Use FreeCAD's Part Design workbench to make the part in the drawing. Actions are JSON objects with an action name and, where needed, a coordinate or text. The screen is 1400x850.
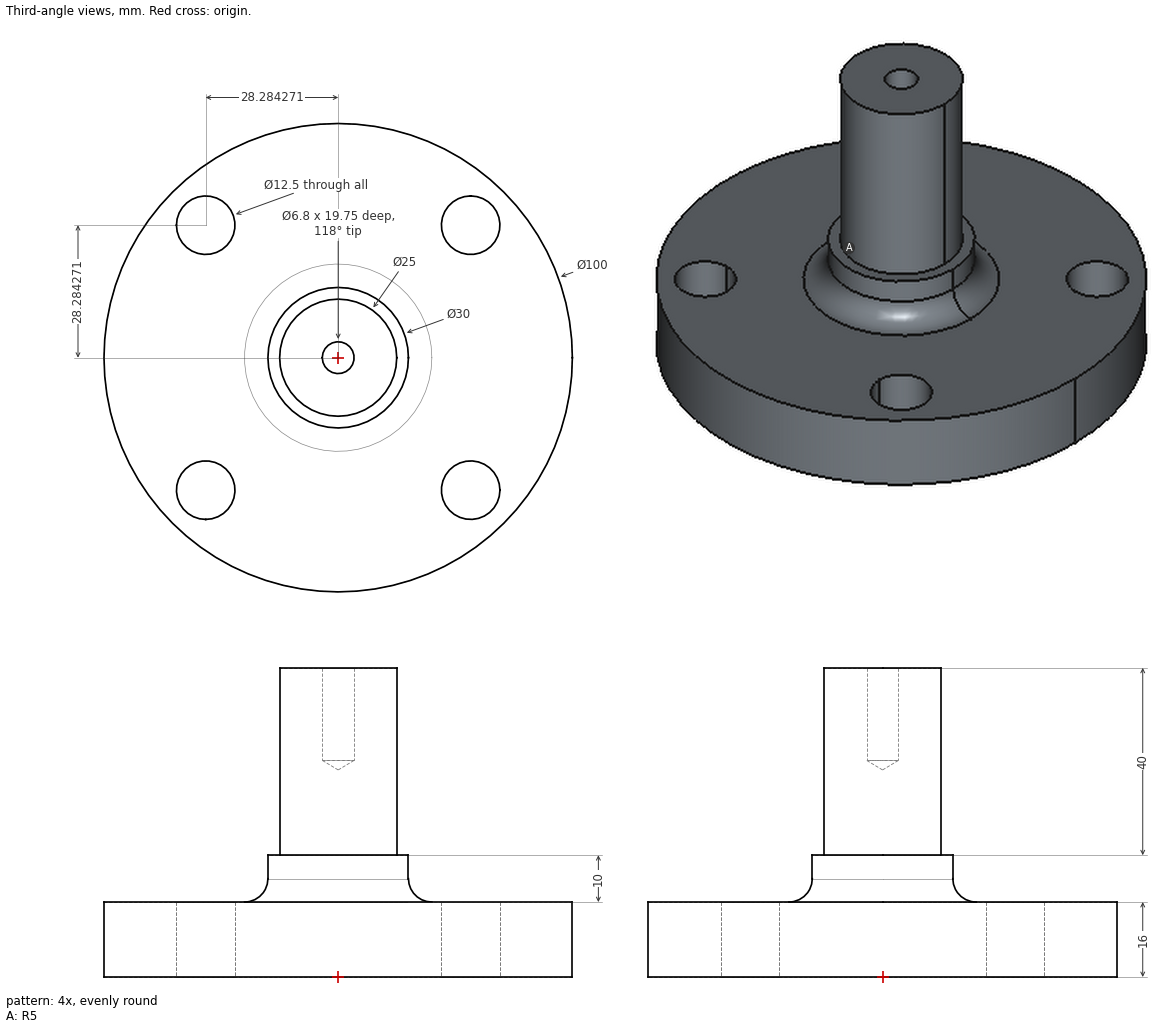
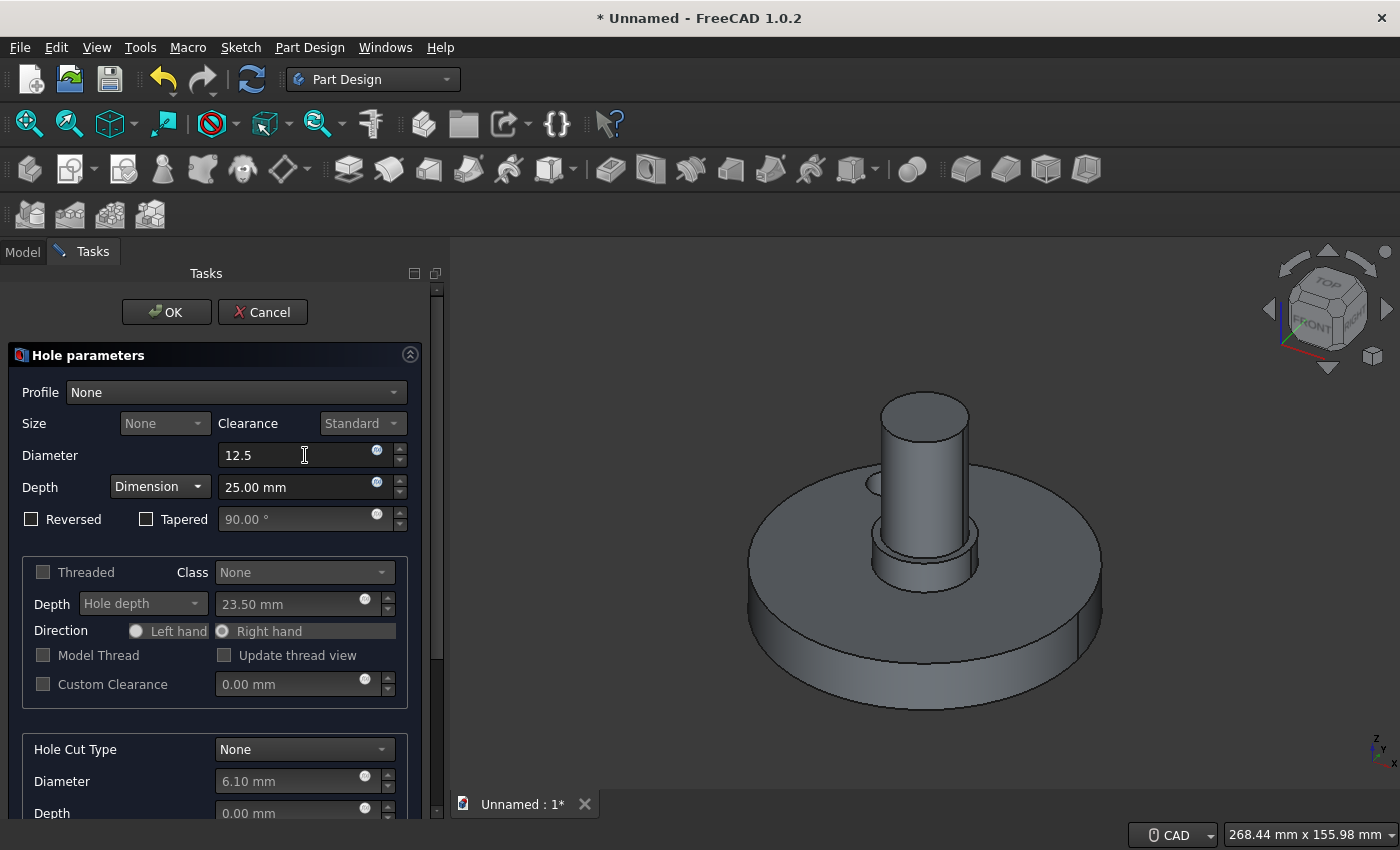
{"action": "left_click", "coordinate": [161, 486]}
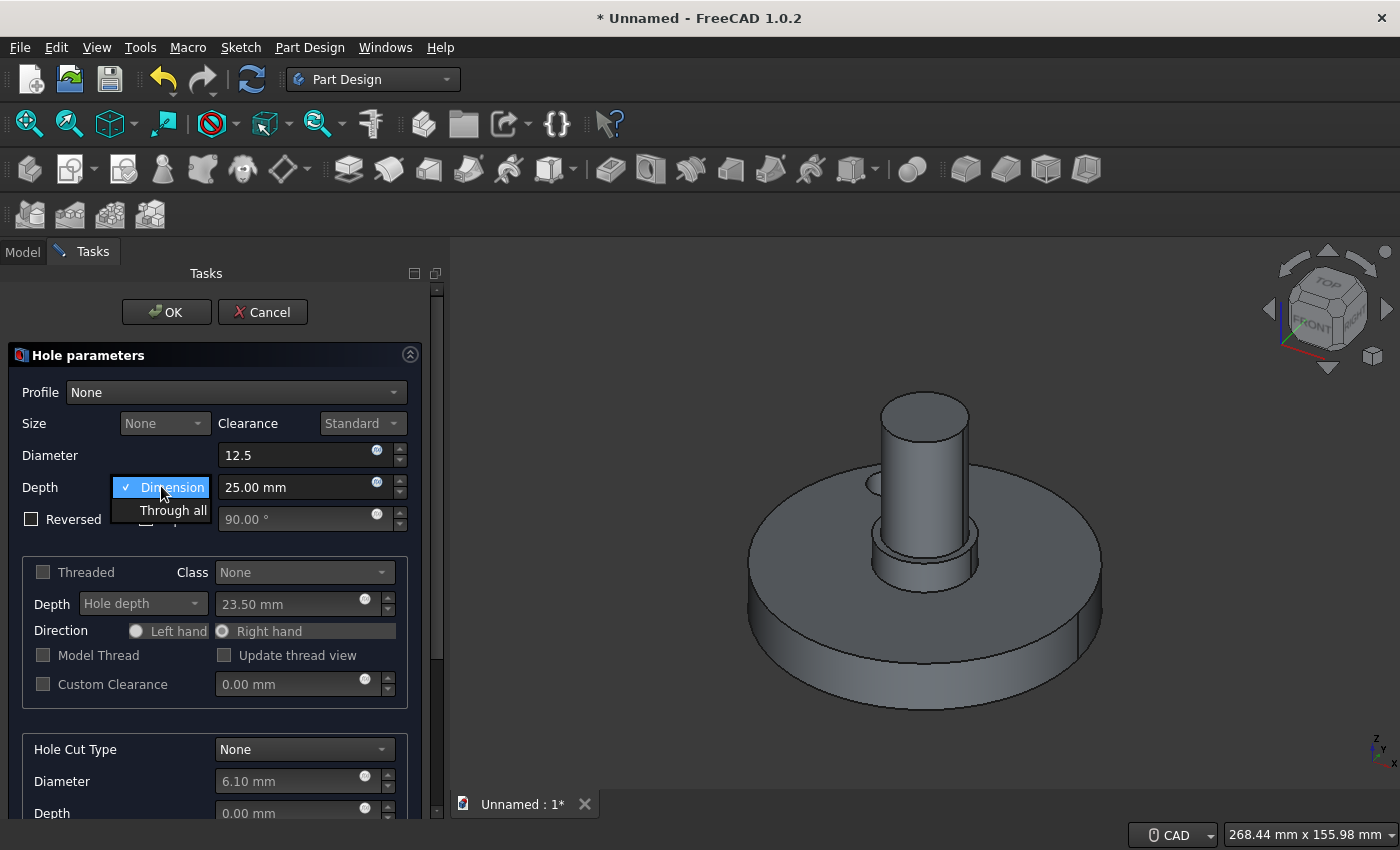
{"action": "left_click", "coordinate": [160, 510]}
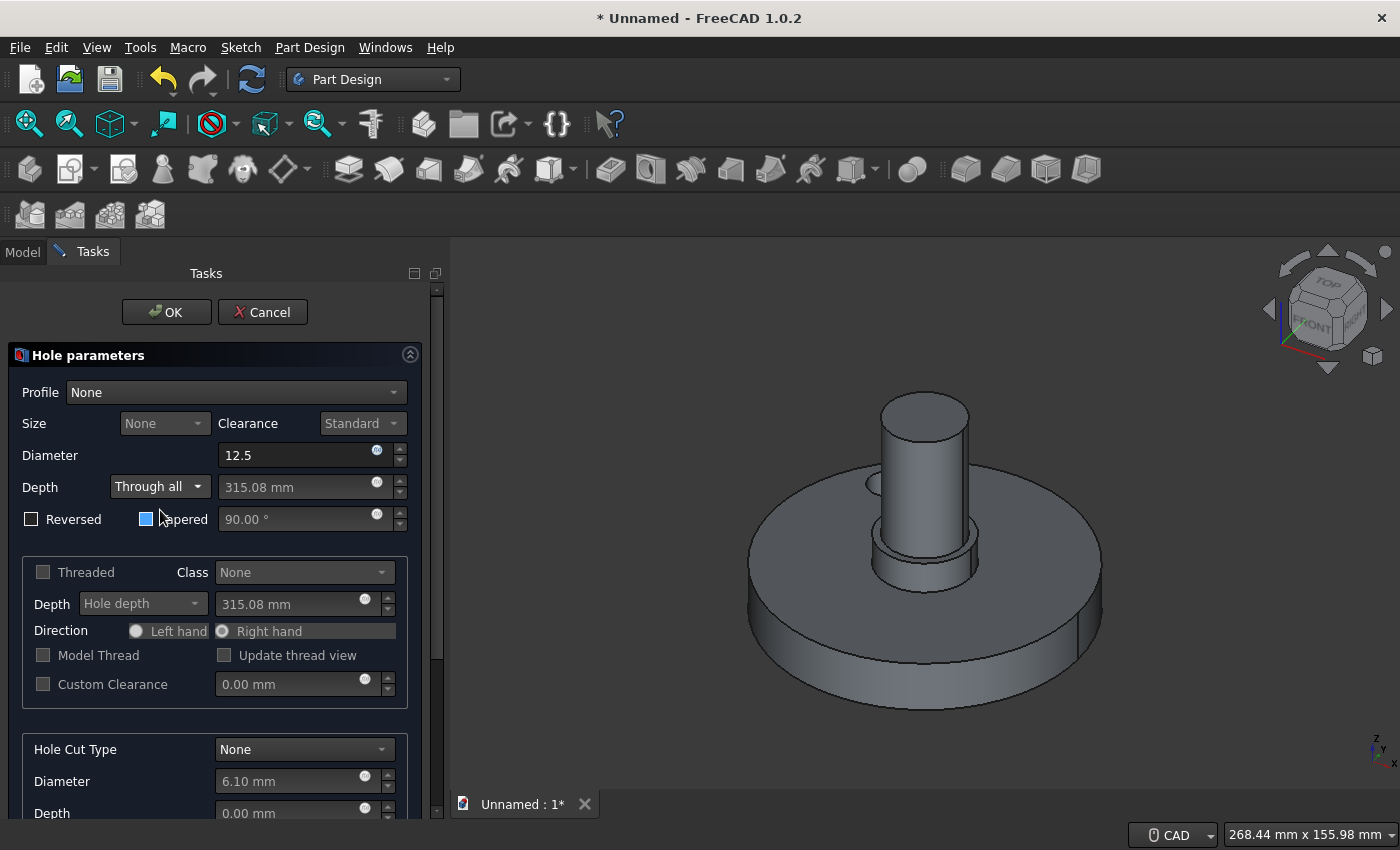
{"action": "left_click", "coordinate": [167, 312]}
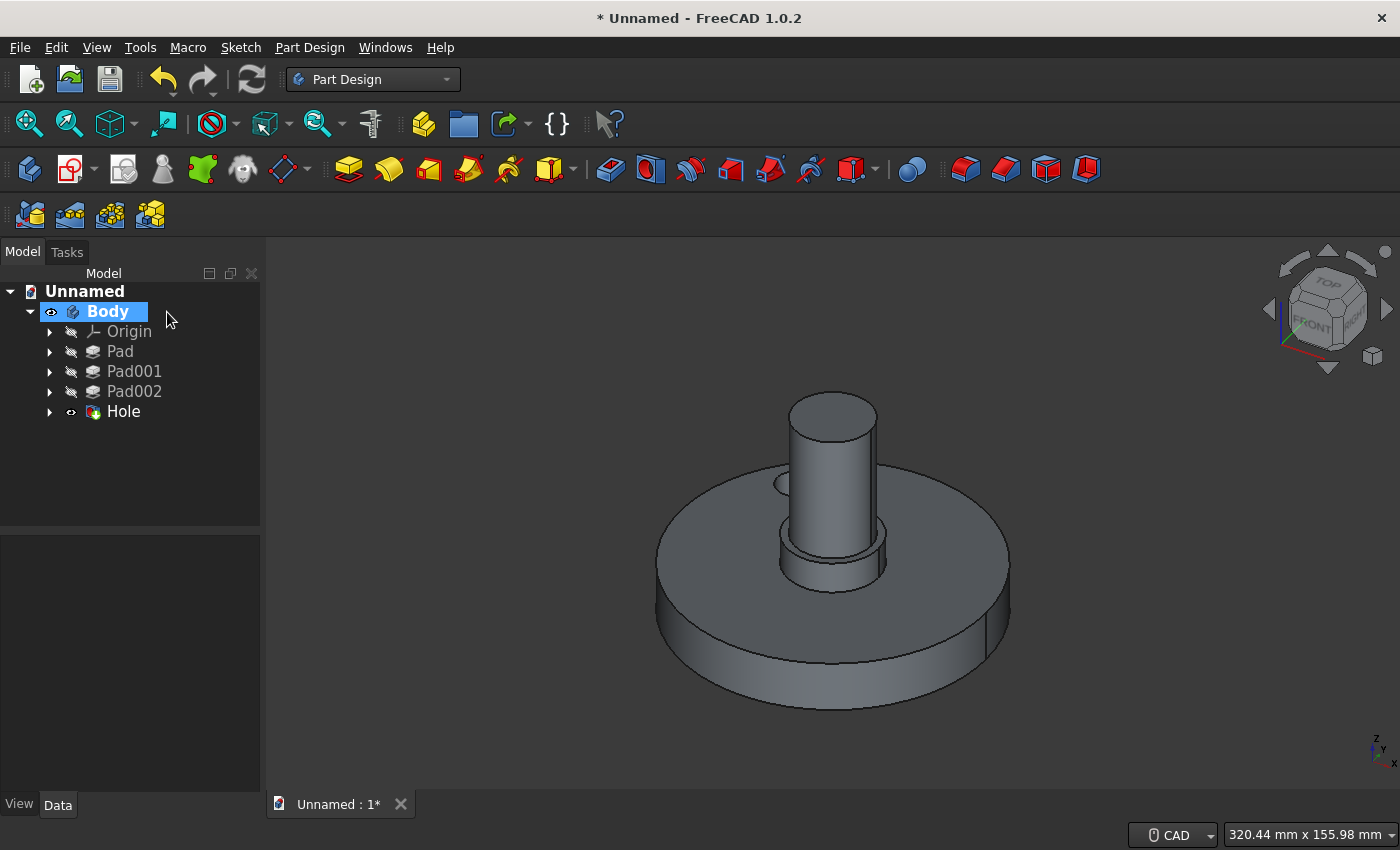
{"action": "left_click", "coordinate": [116, 412]}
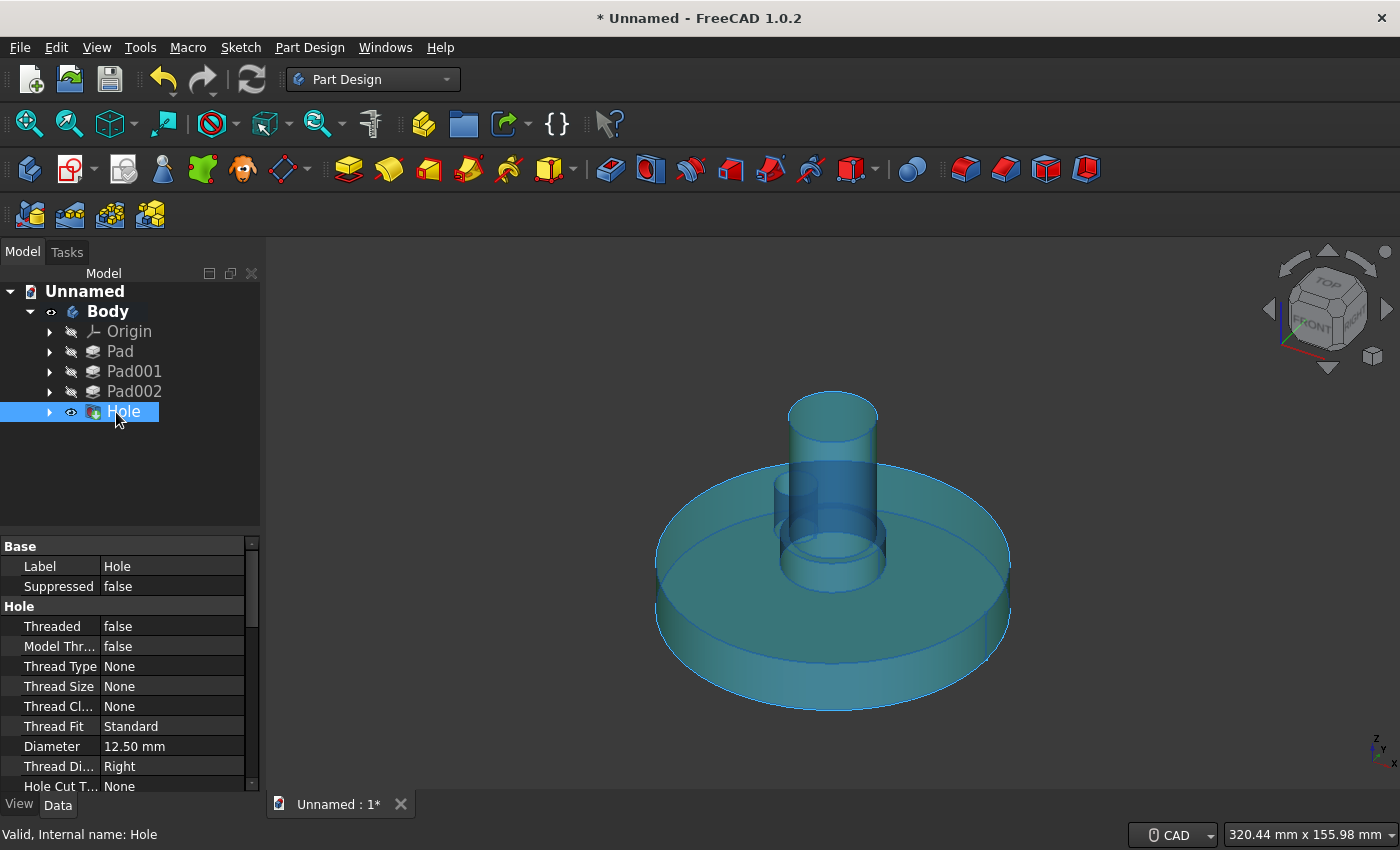
{"action": "left_click", "coordinate": [110, 214]}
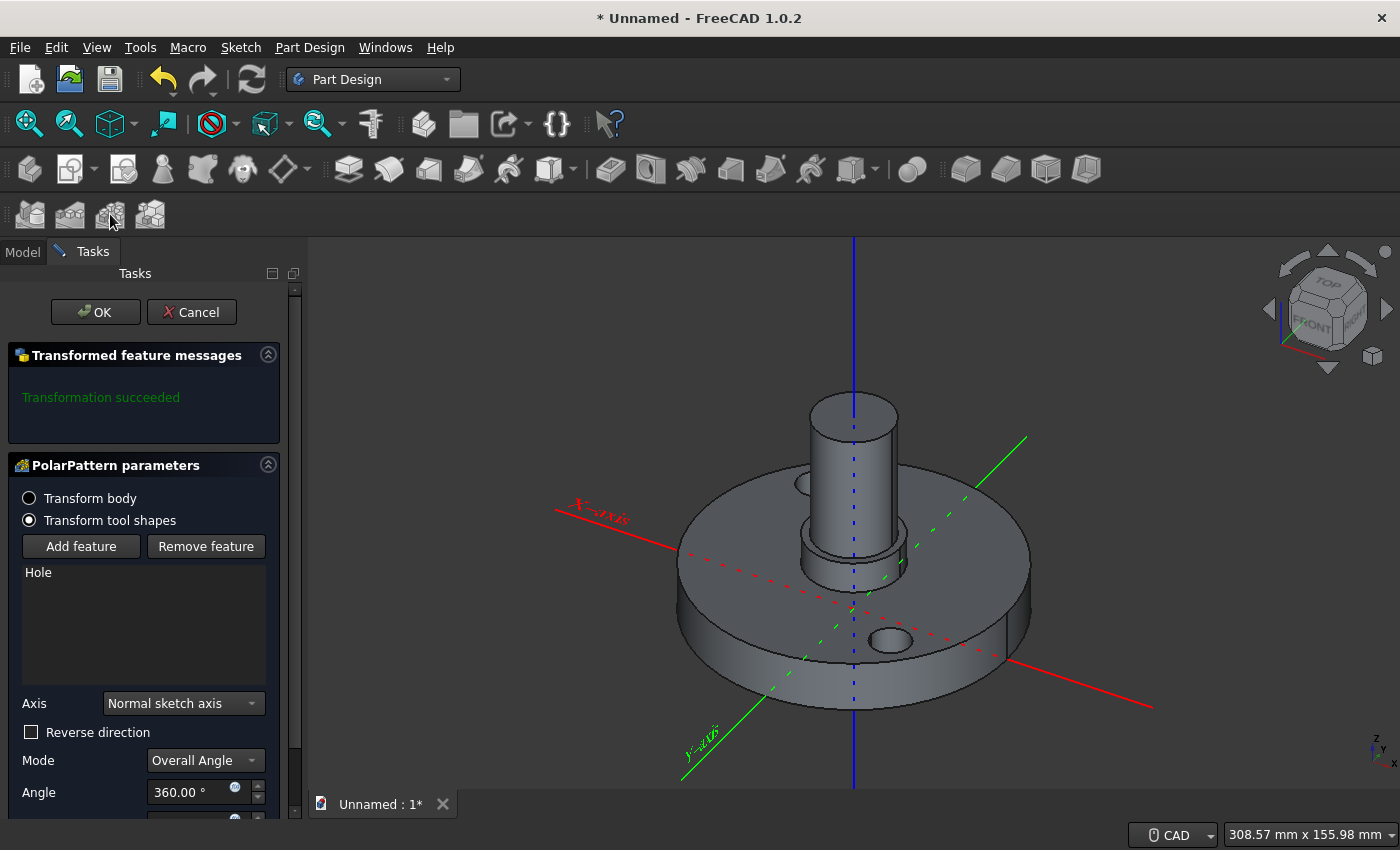
{"action": "left_click", "coordinate": [184, 704]}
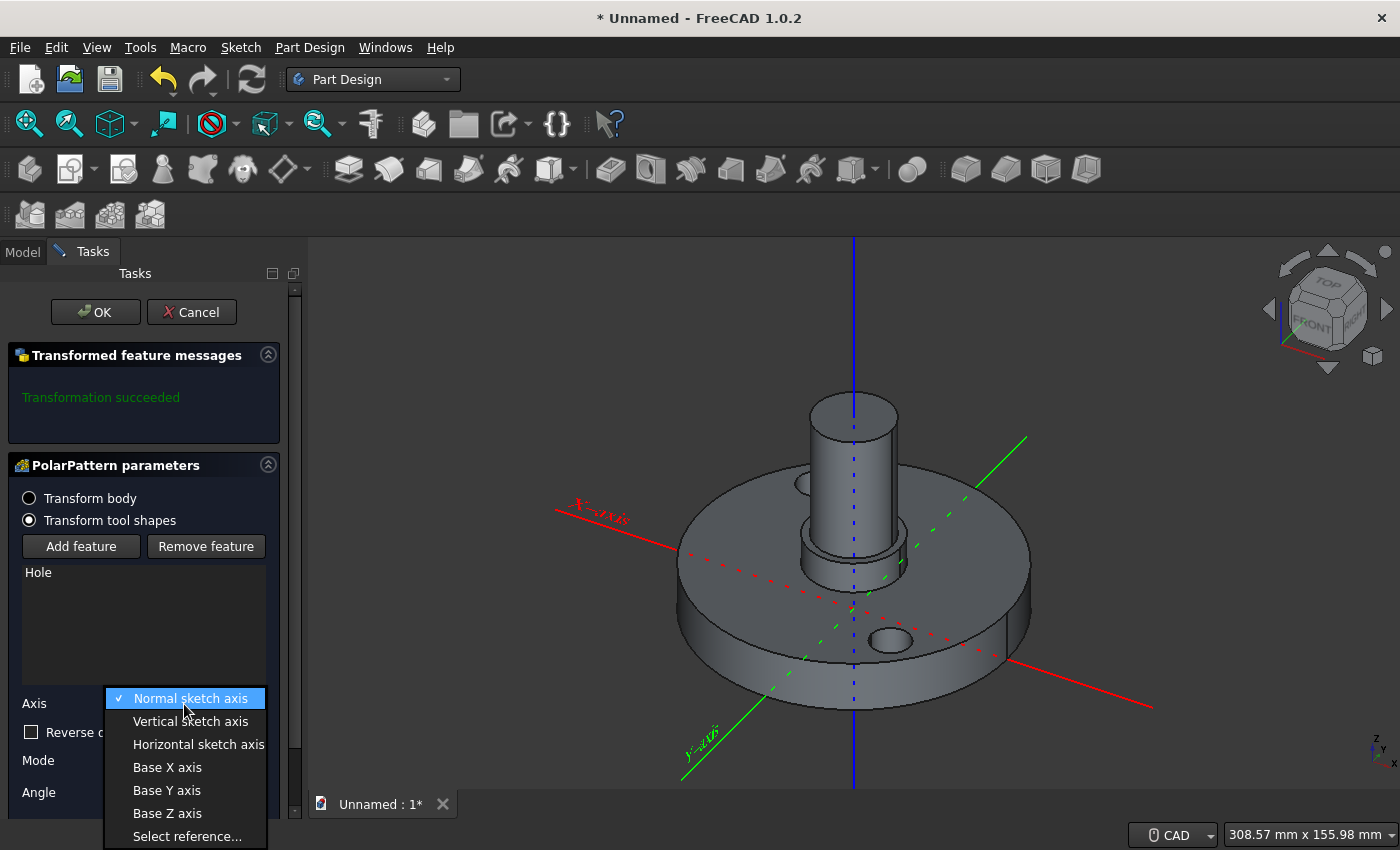
{"action": "left_click", "coordinate": [184, 814]}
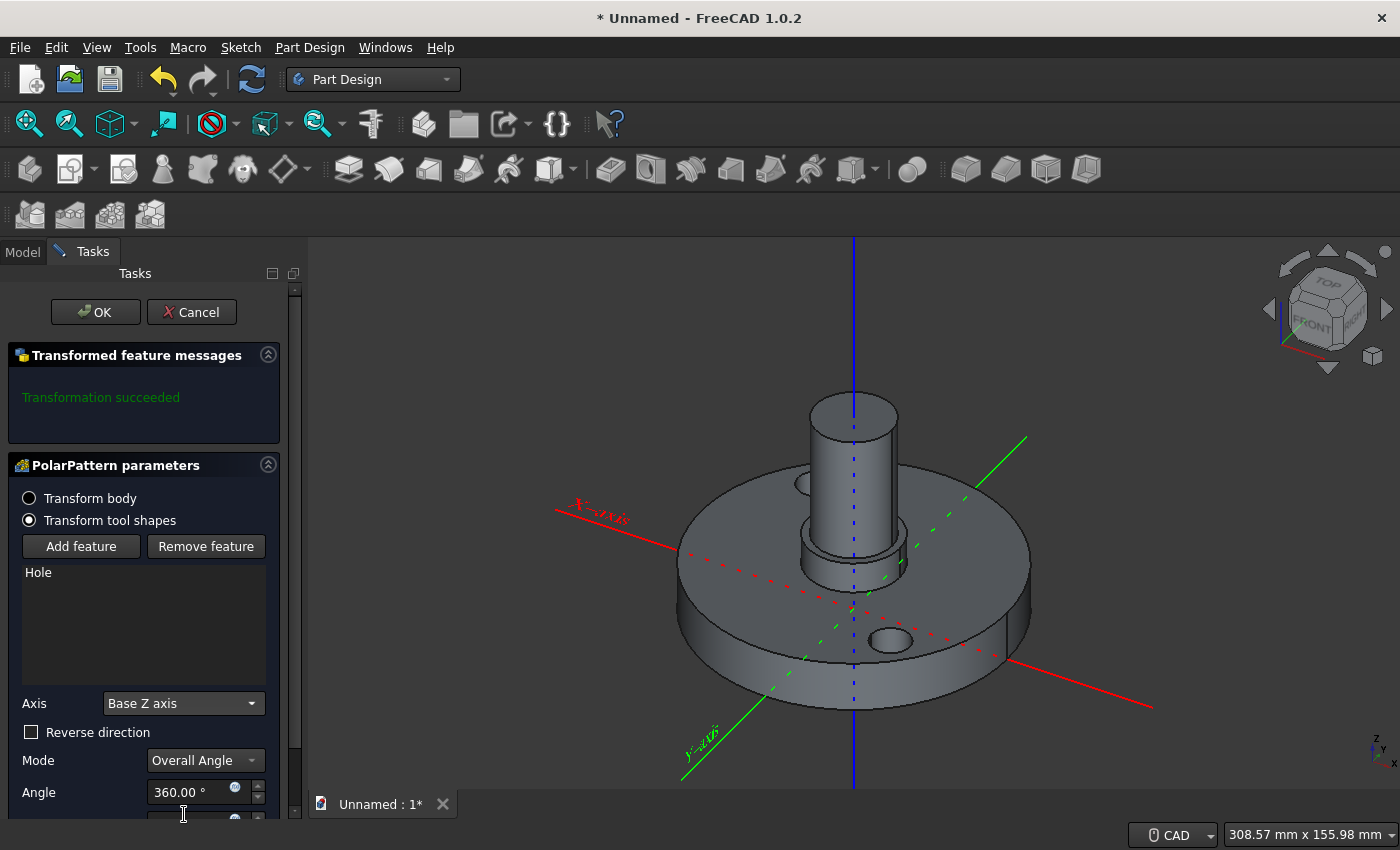
{"action": "scroll", "coordinate": [295, 550], "scroll_direction": "down", "scroll_amount": 2}